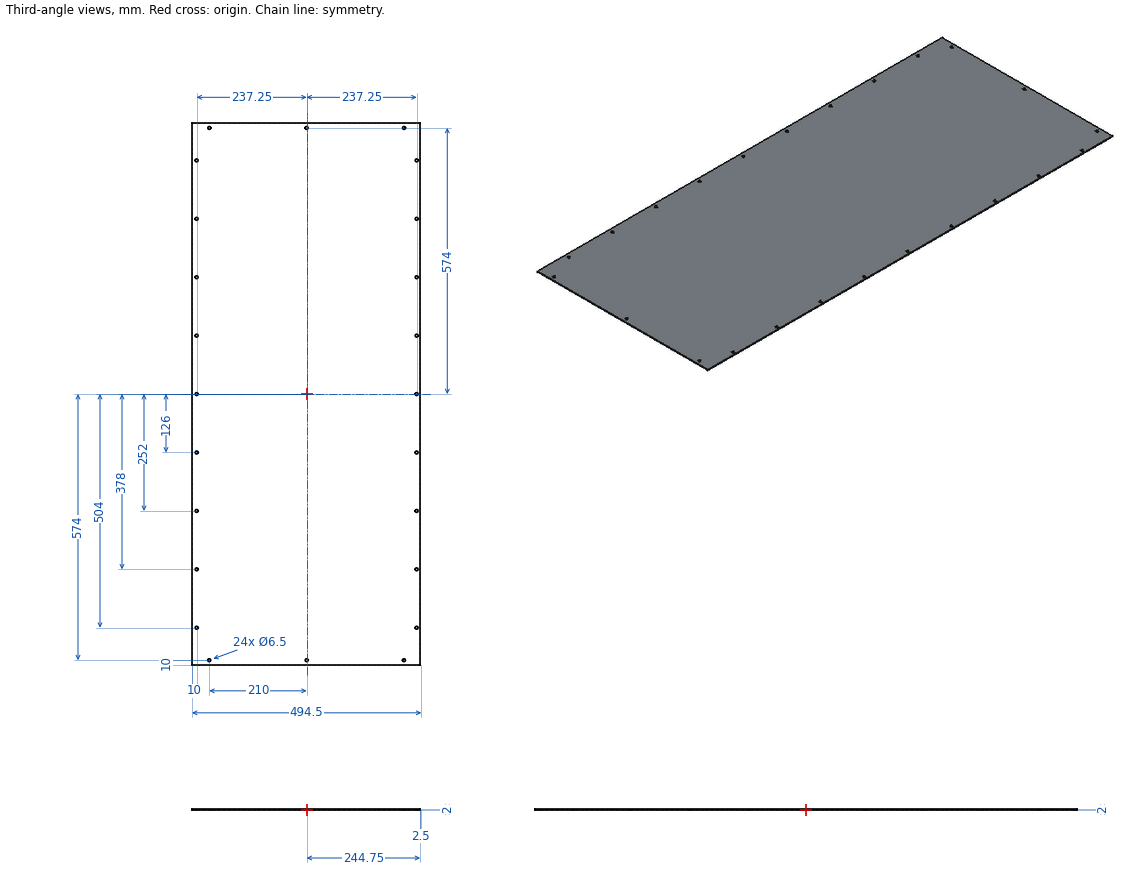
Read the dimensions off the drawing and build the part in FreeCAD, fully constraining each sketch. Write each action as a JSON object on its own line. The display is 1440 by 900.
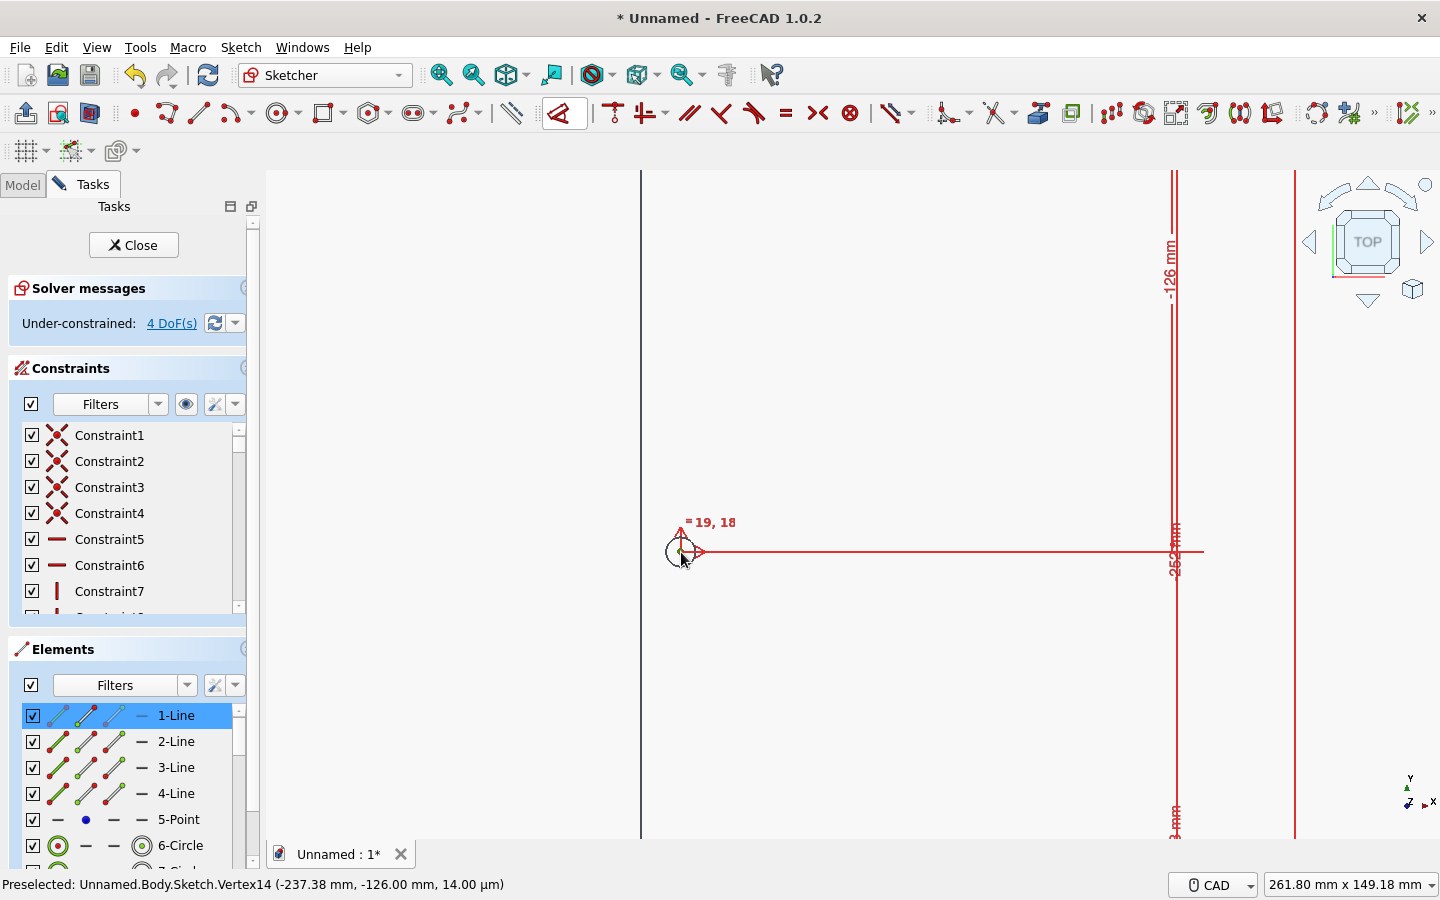
{"action": "key", "text": "l"}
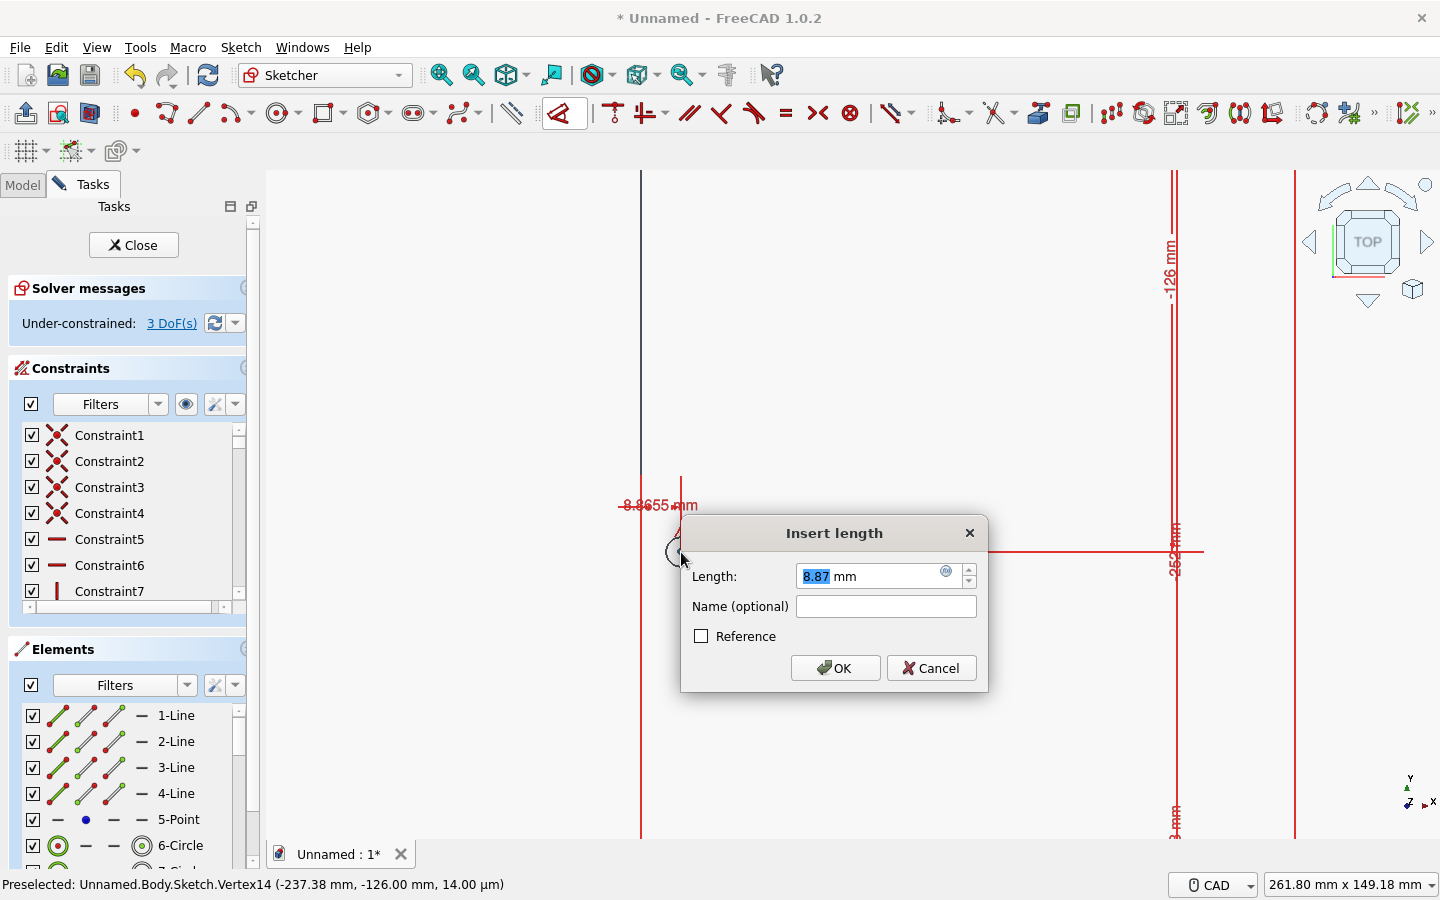
{"action": "type", "text": "10"}
{"action": "key", "text": "Return"}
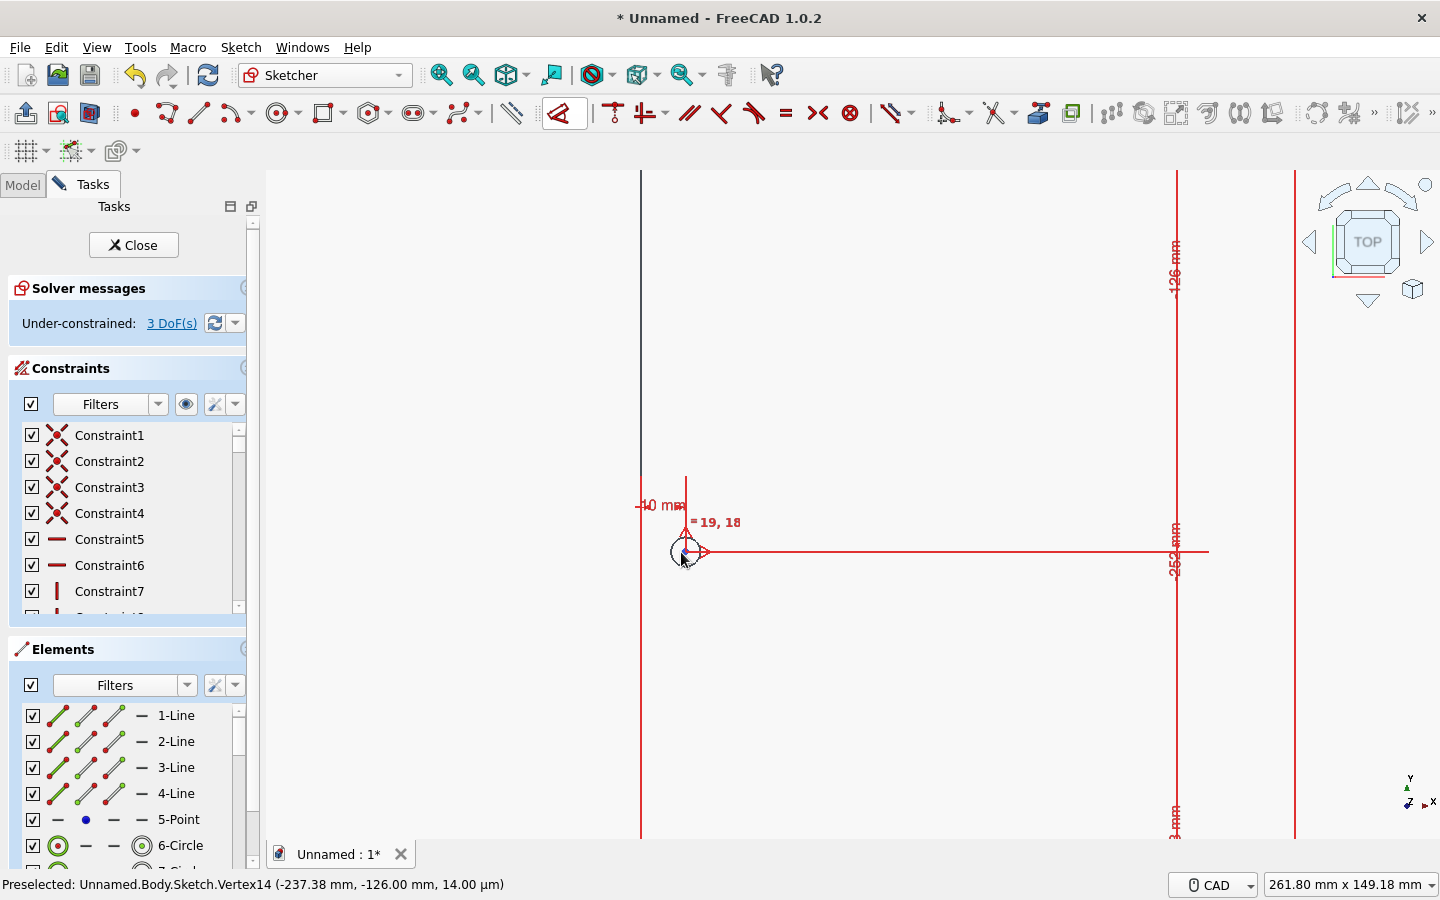
{"action": "scroll", "coordinate": [689, 556], "scroll_direction": "down", "scroll_amount": 12}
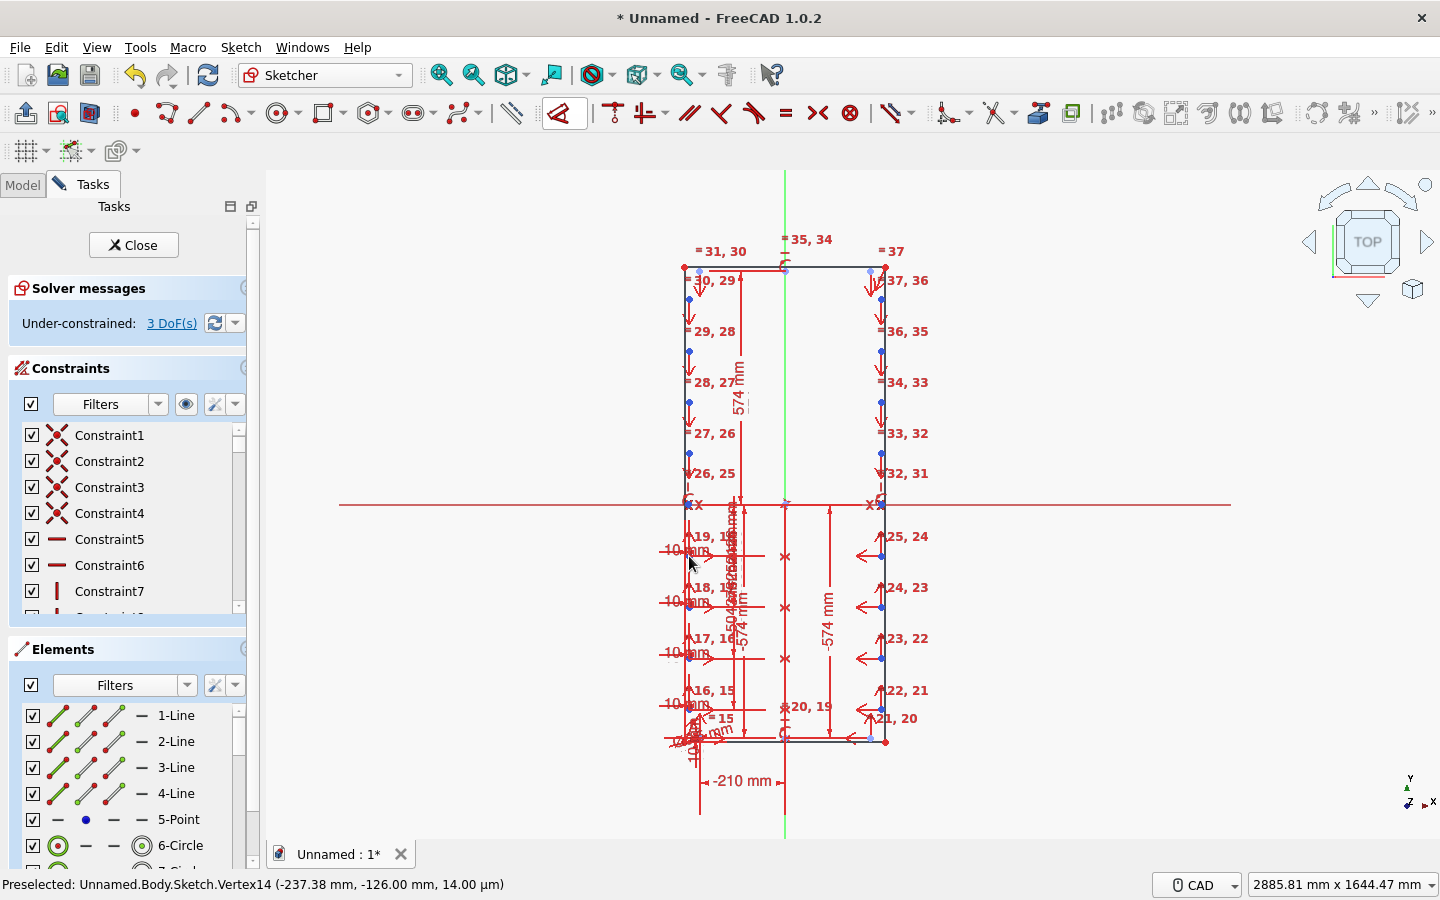
{"action": "left_click", "coordinate": [745, 742]}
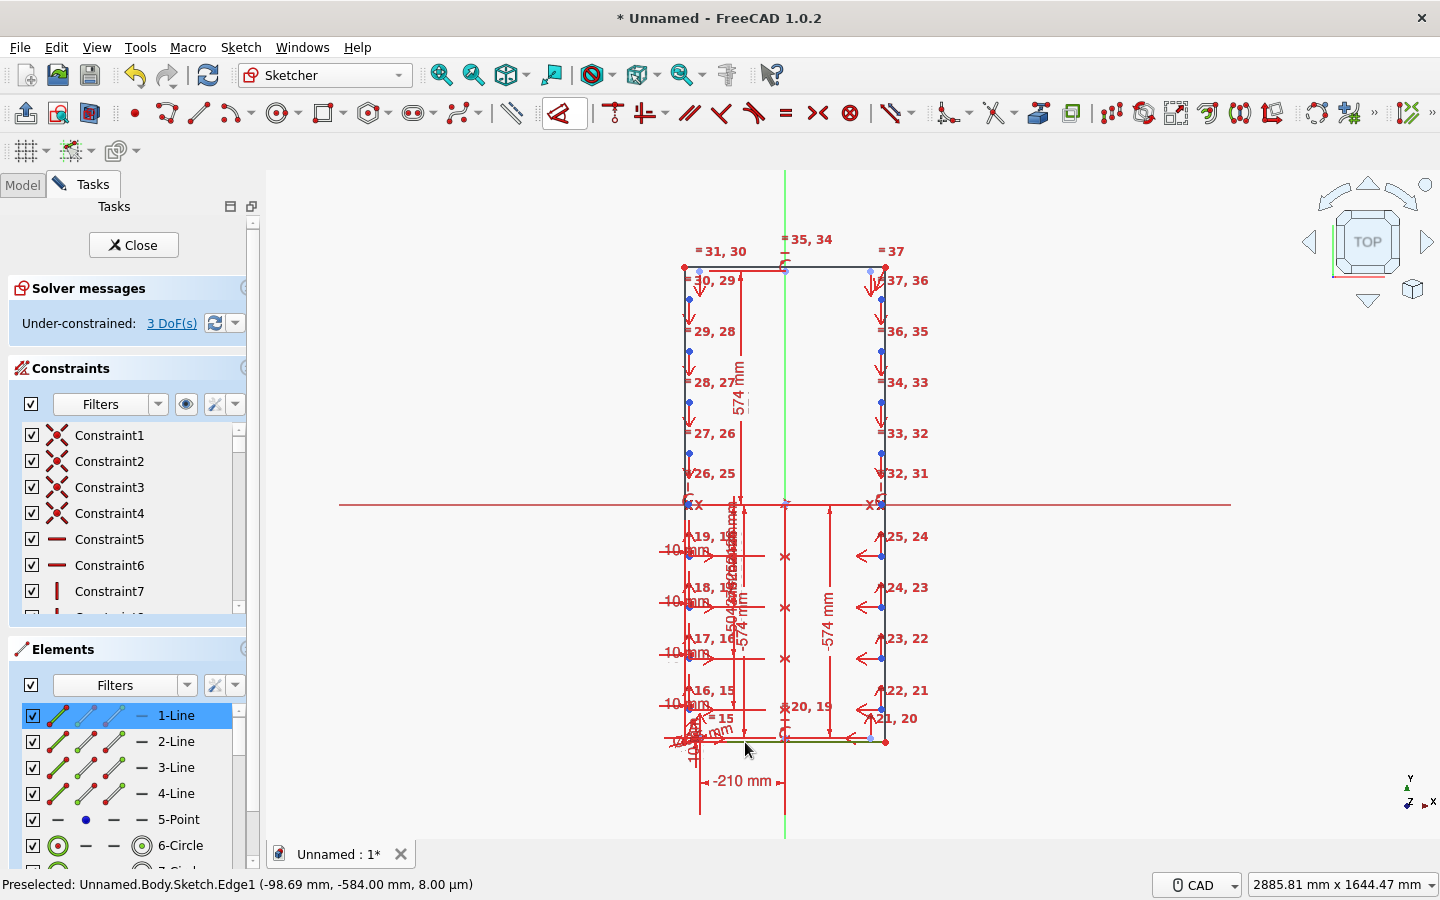
{"action": "left_click", "coordinate": [582, 114]}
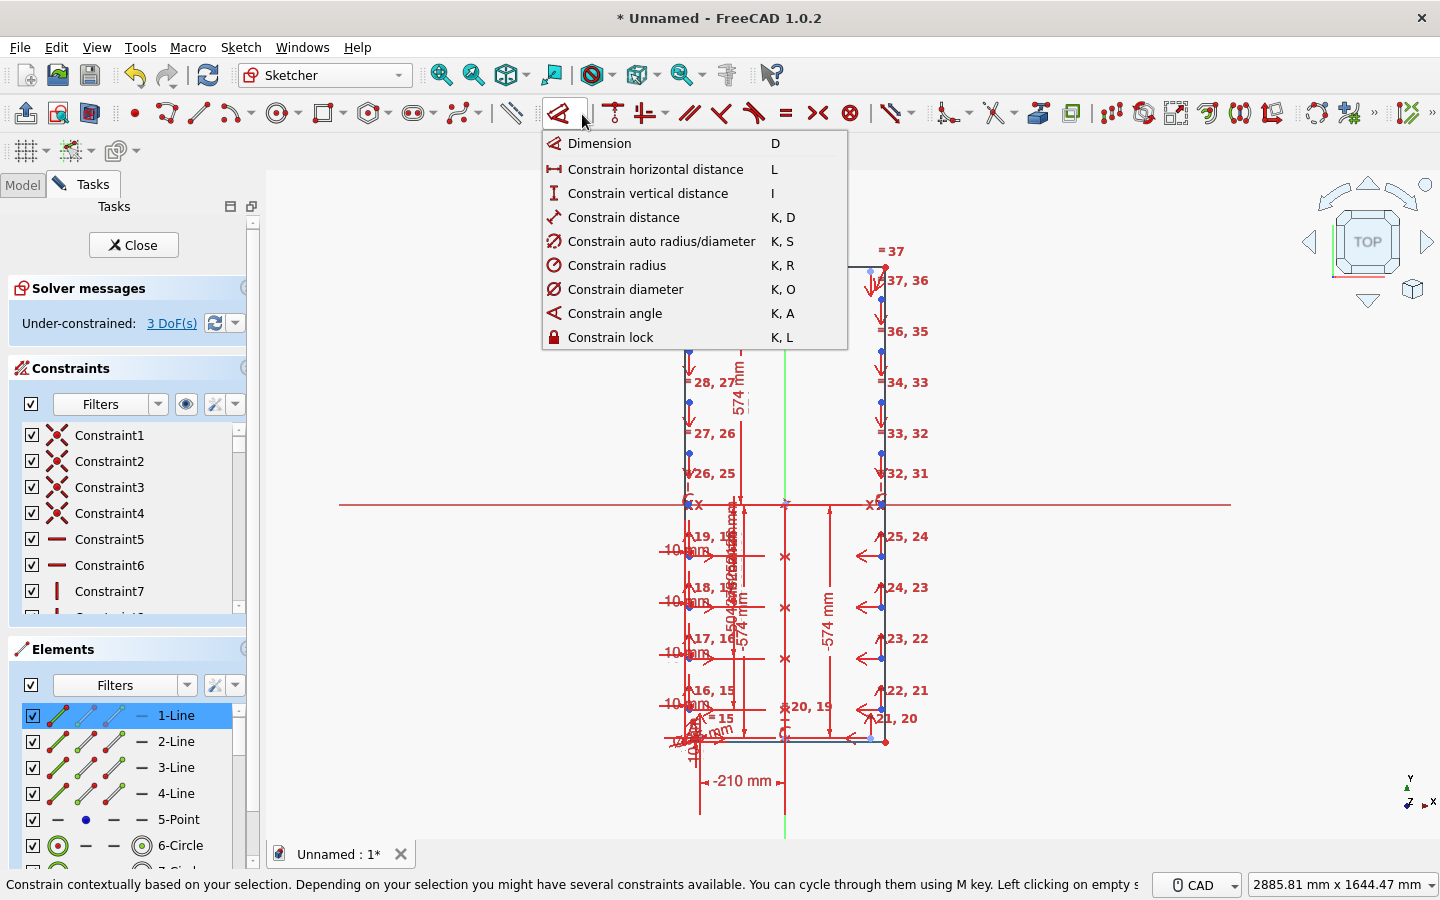
{"action": "left_click", "coordinate": [695, 169]}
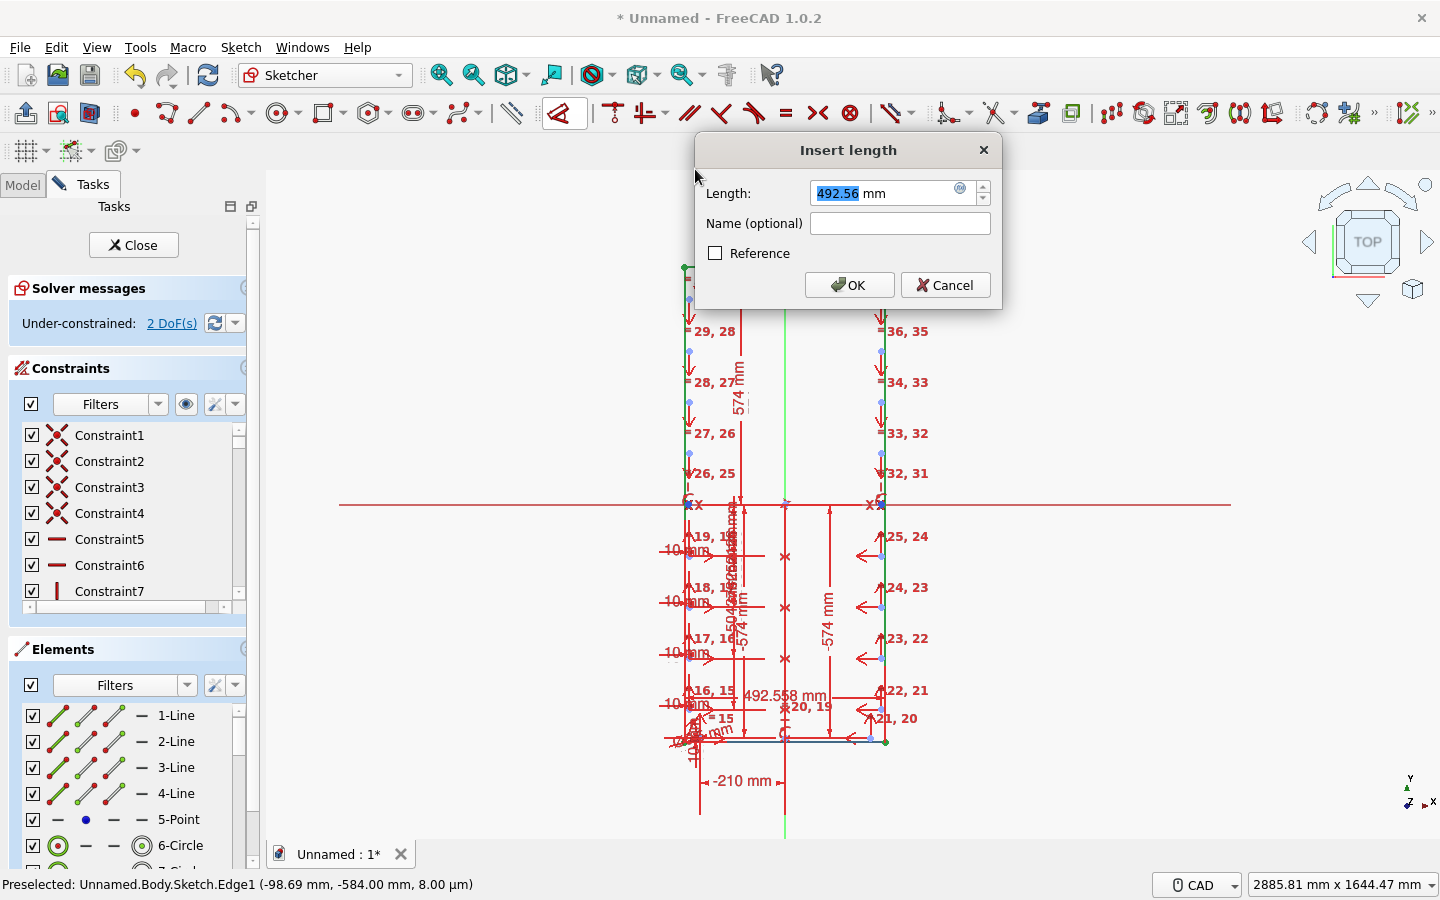
{"action": "type", "text": "494.5"}
{"action": "key", "text": "Return"}